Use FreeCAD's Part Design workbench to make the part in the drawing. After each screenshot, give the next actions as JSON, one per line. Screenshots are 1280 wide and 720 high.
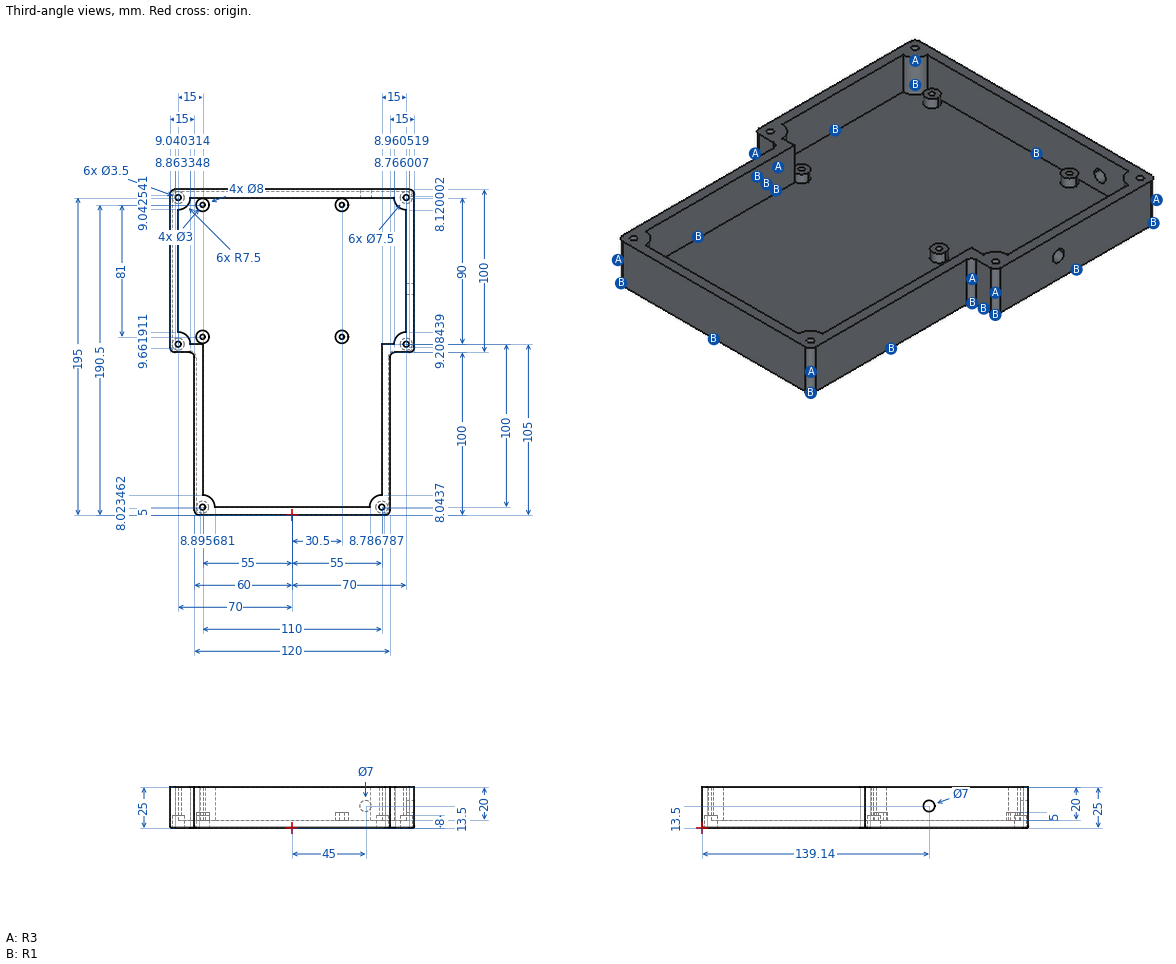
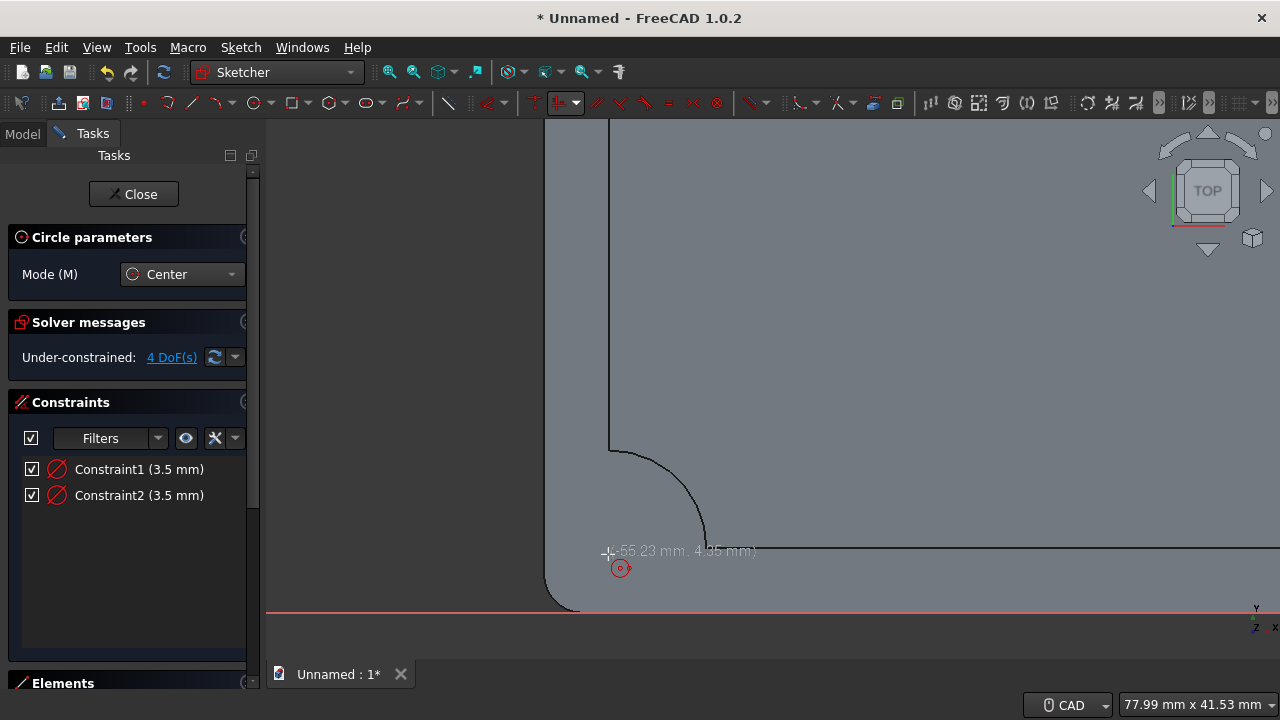
{"action": "scroll", "coordinate": [608, 554], "scroll_direction": "down", "scroll_amount": 10}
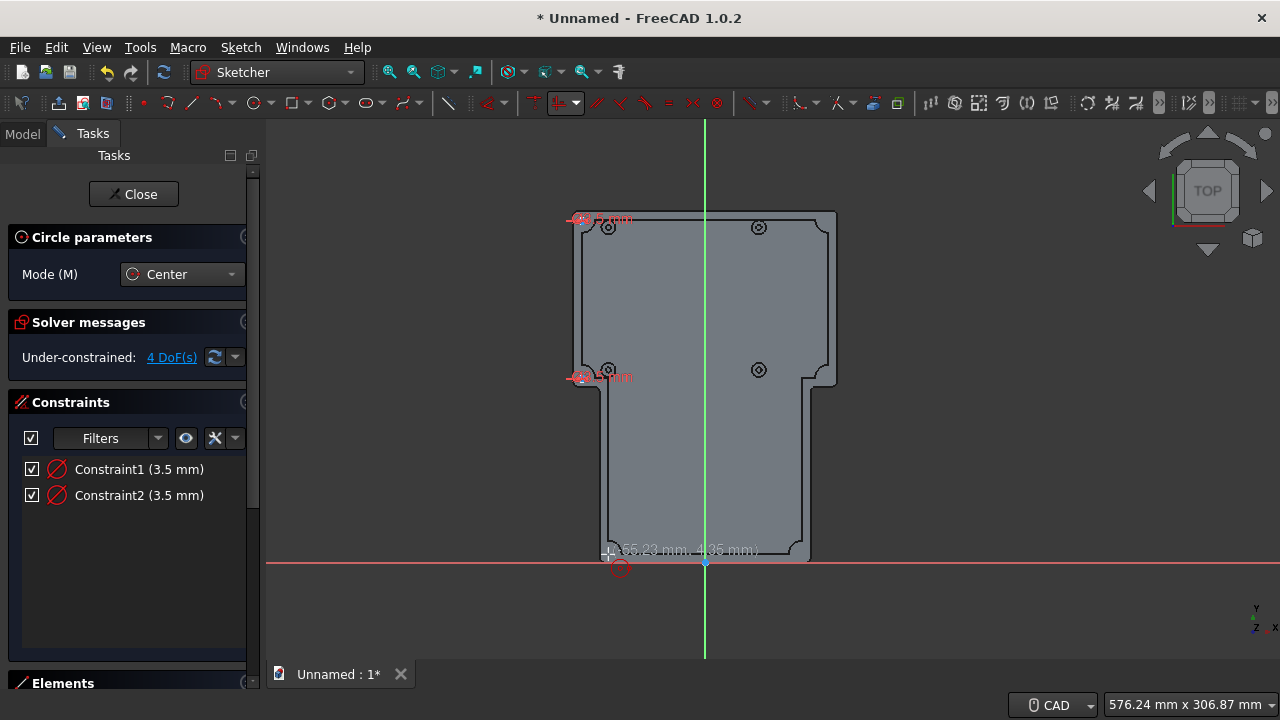
{"action": "scroll", "coordinate": [608, 554], "scroll_direction": "up", "scroll_amount": 3}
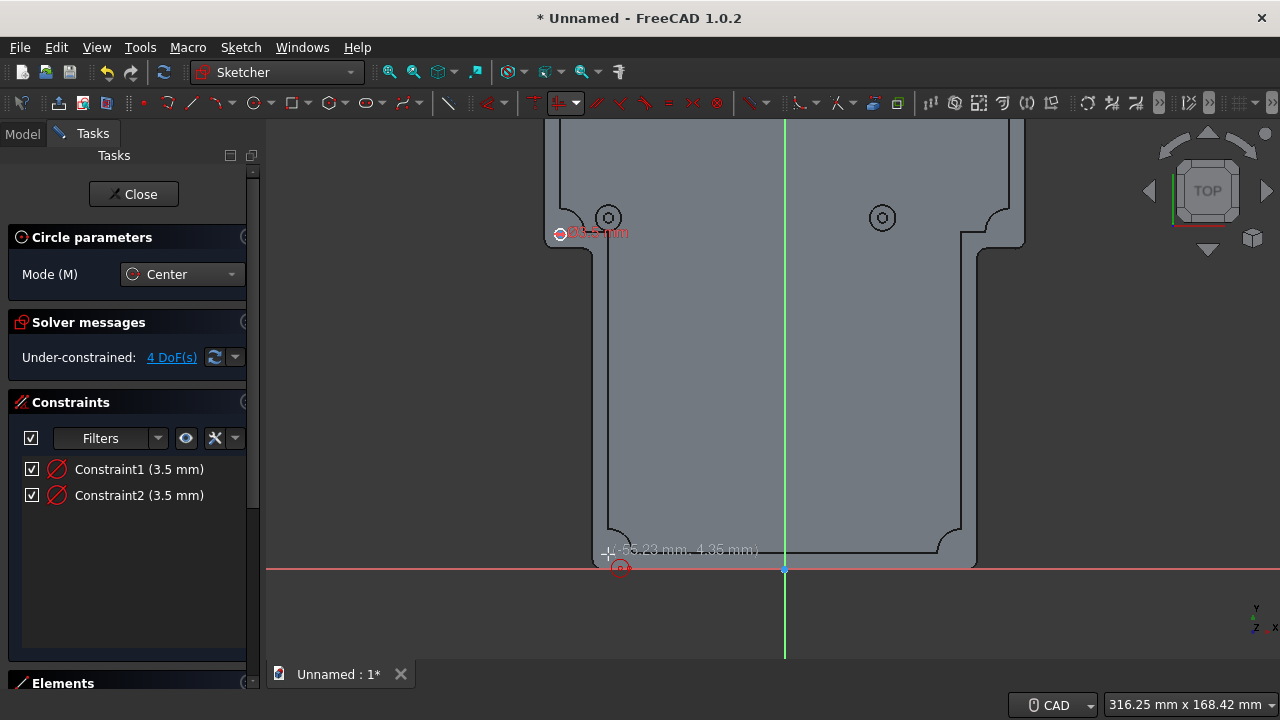
{"action": "left_click", "coordinate": [608, 553]}
{"action": "mouse_move", "coordinate": [612, 549]}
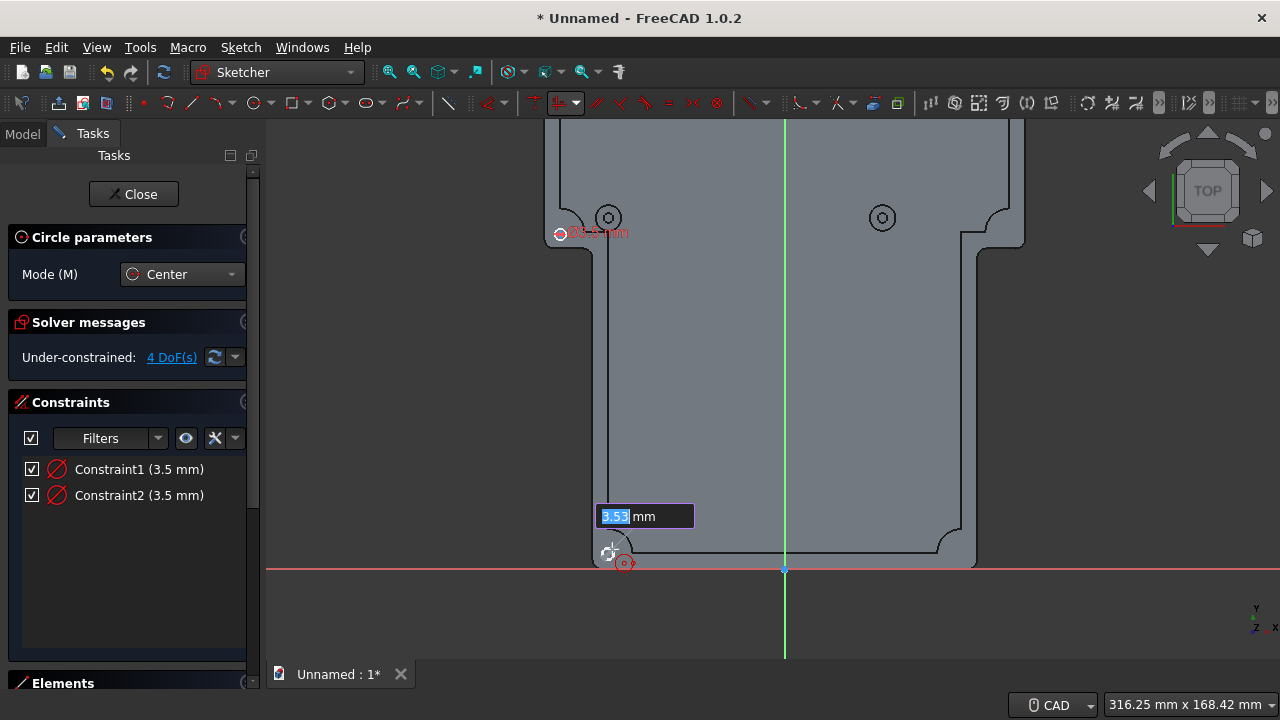
{"action": "type", "text": "3.5"}
{"action": "key", "text": "Return"}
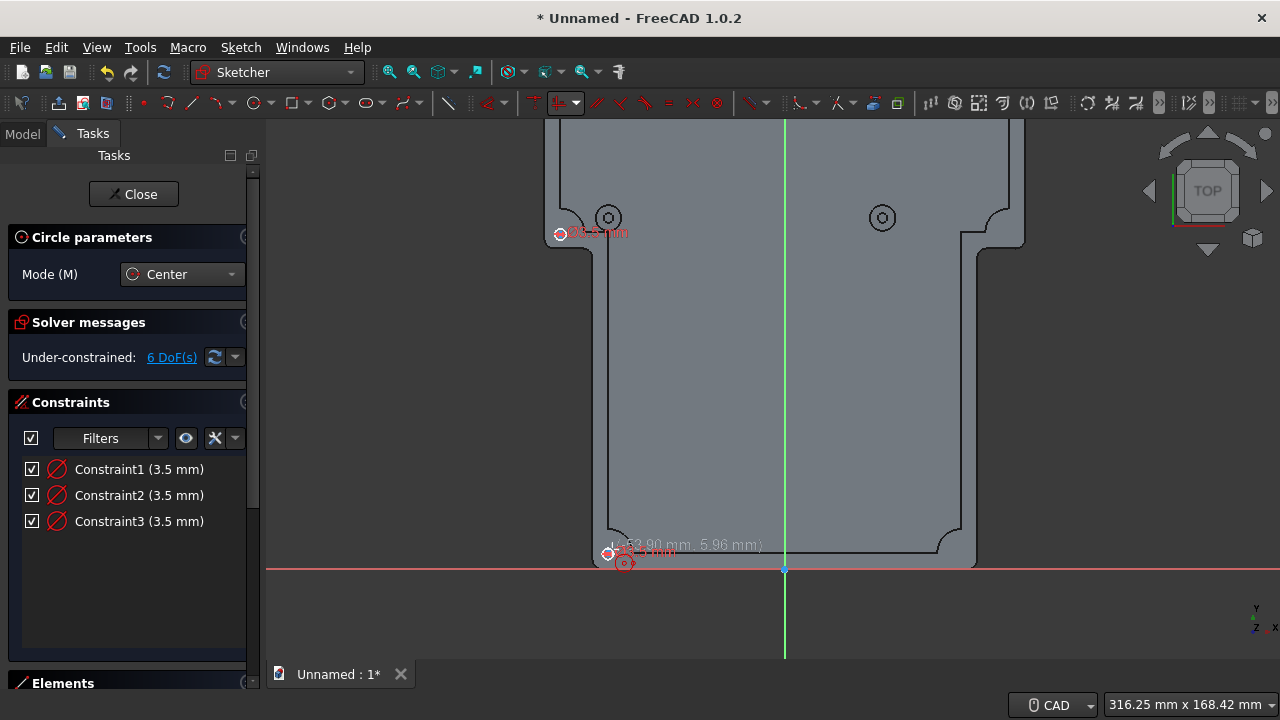
{"action": "scroll", "coordinate": [961, 553], "scroll_direction": "up", "scroll_amount": 7}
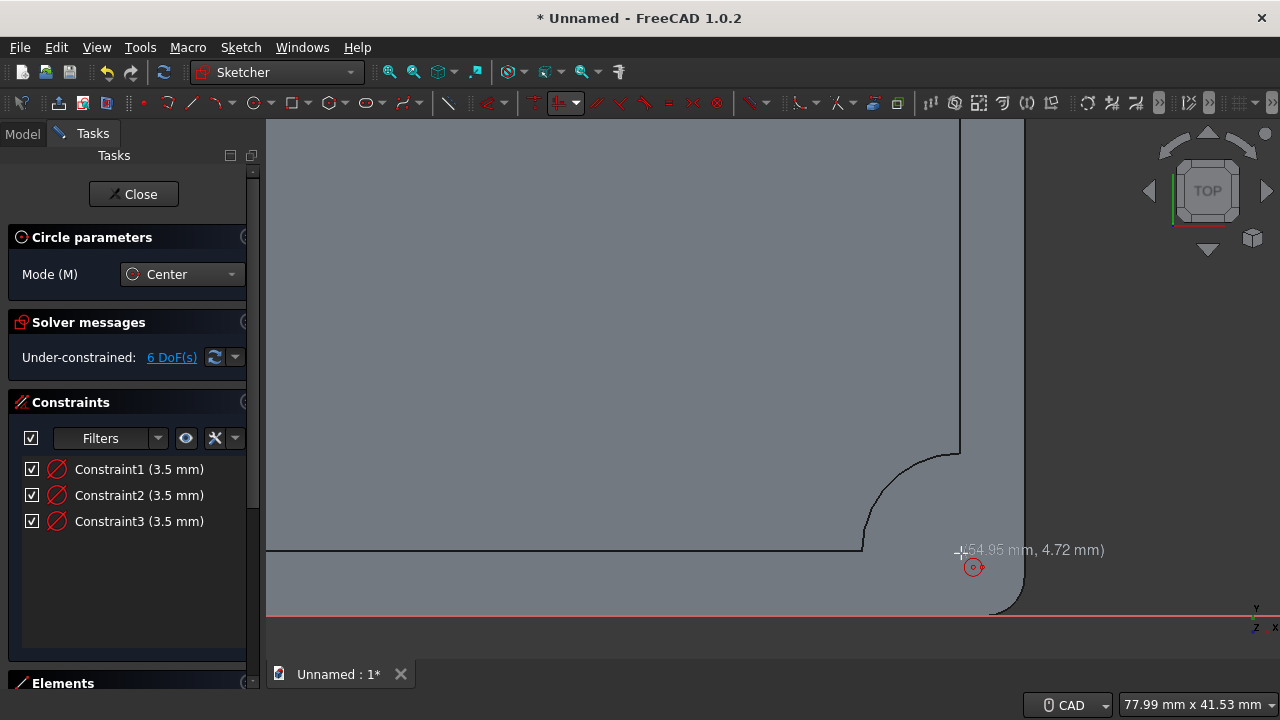
{"action": "scroll", "coordinate": [777, 554], "scroll_direction": "down", "scroll_amount": 10}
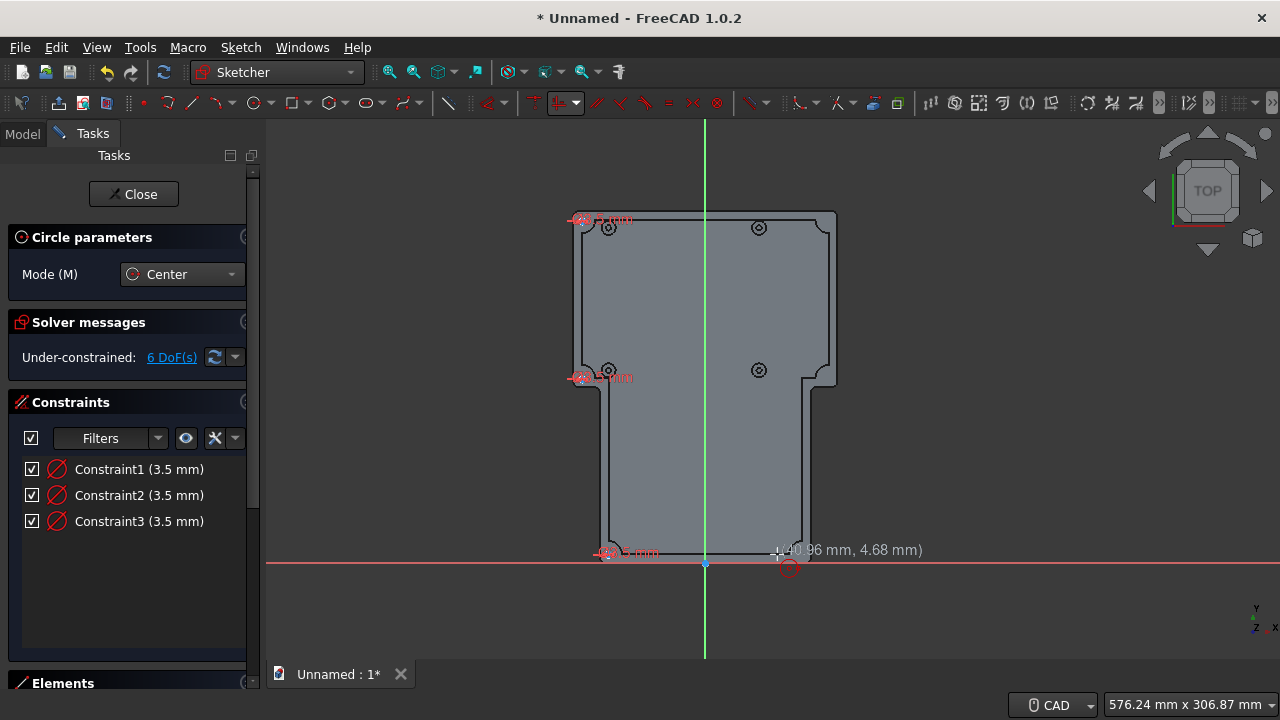
{"action": "scroll", "coordinate": [802, 554], "scroll_direction": "up", "scroll_amount": 3}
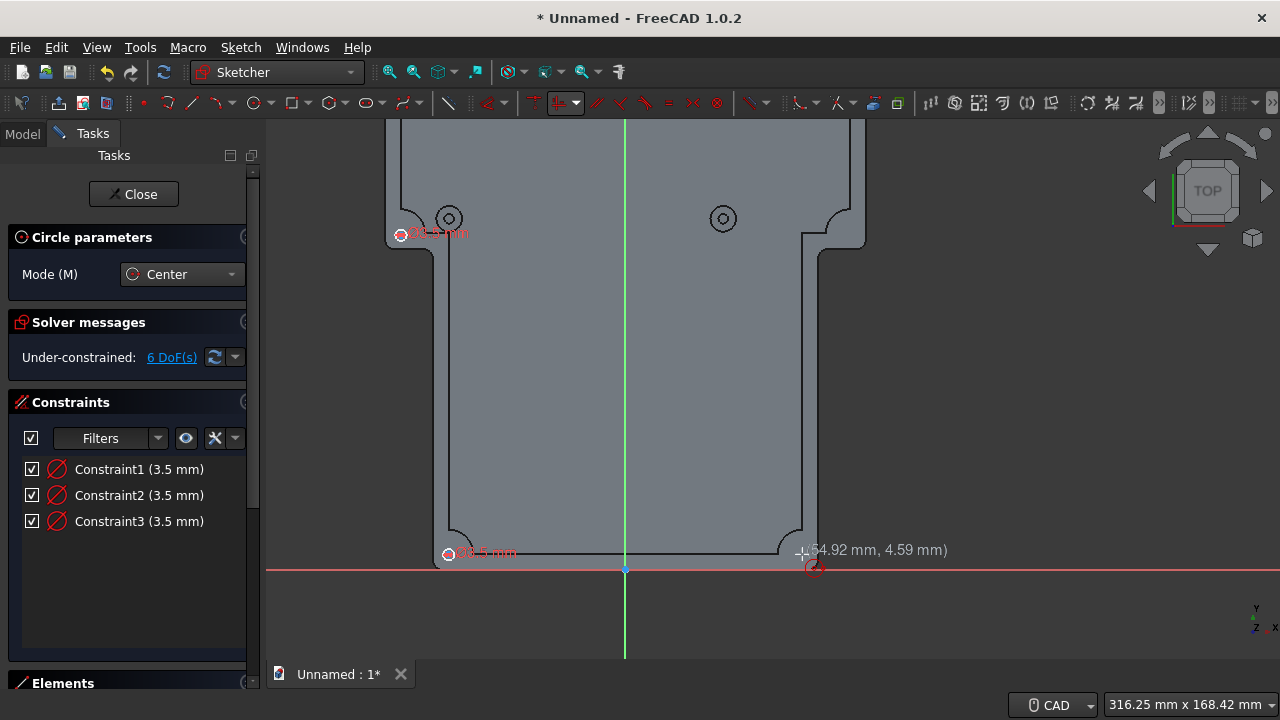
{"action": "left_click", "coordinate": [802, 554]}
{"action": "mouse_move", "coordinate": [806, 550]}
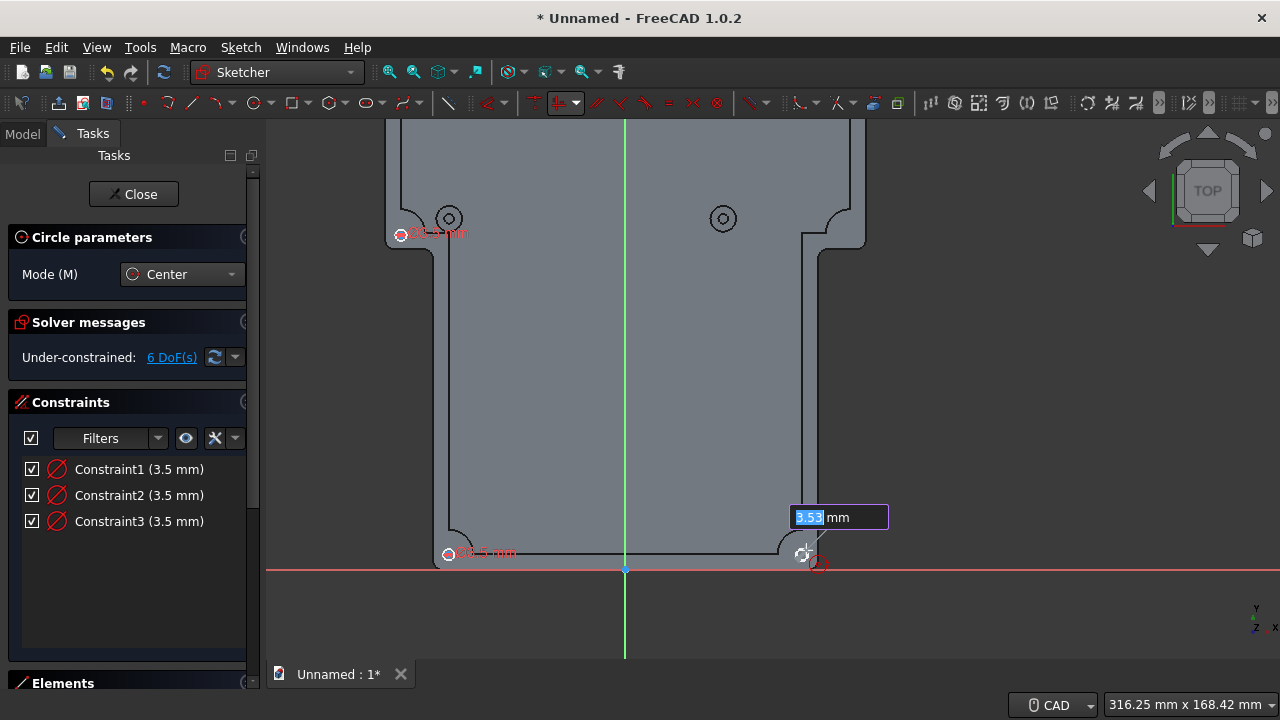
{"action": "type", "text": "3.5"}
{"action": "key", "text": "Return"}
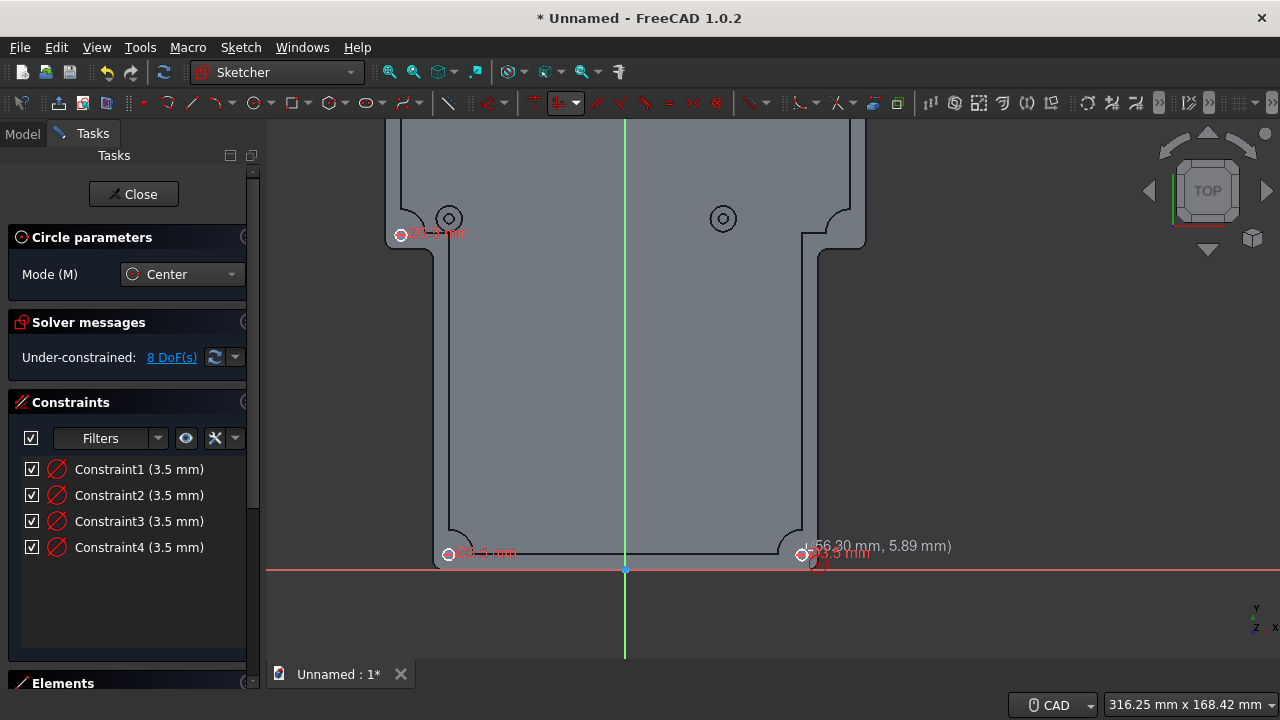
{"action": "scroll", "coordinate": [850, 233], "scroll_direction": "up", "scroll_amount": 7}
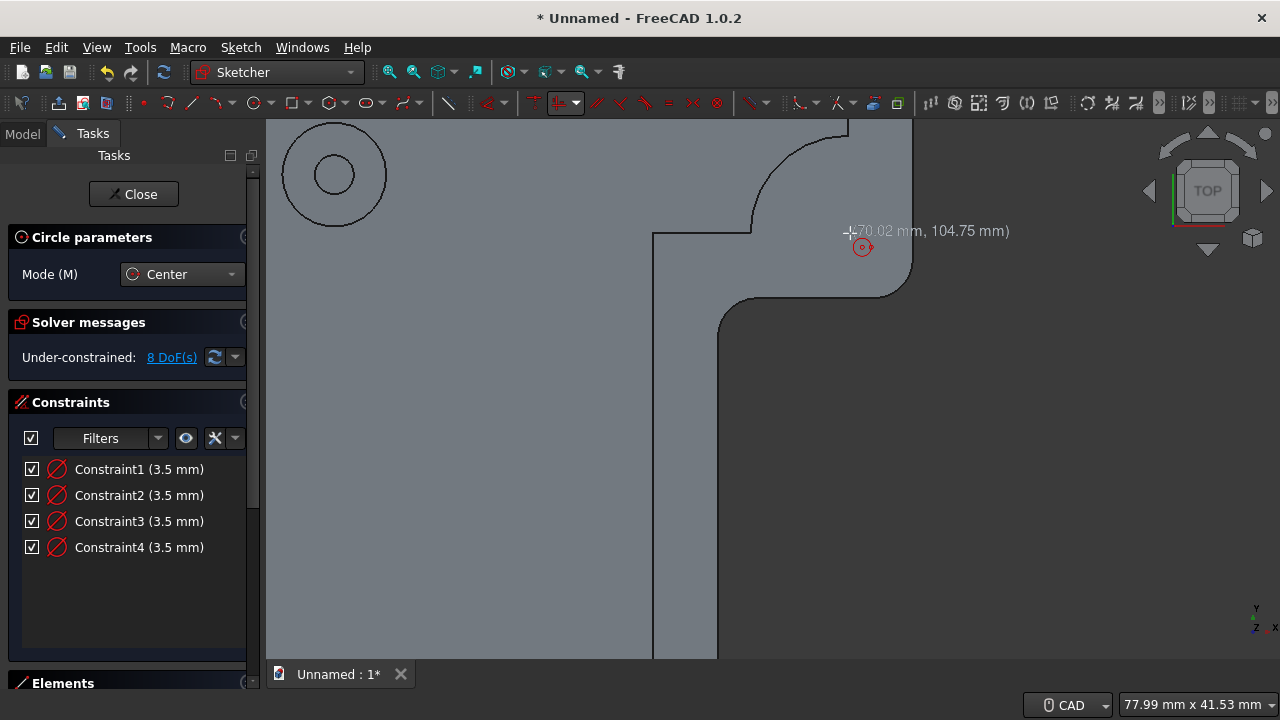
{"action": "scroll", "coordinate": [825, 400], "scroll_direction": "down", "scroll_amount": 10}